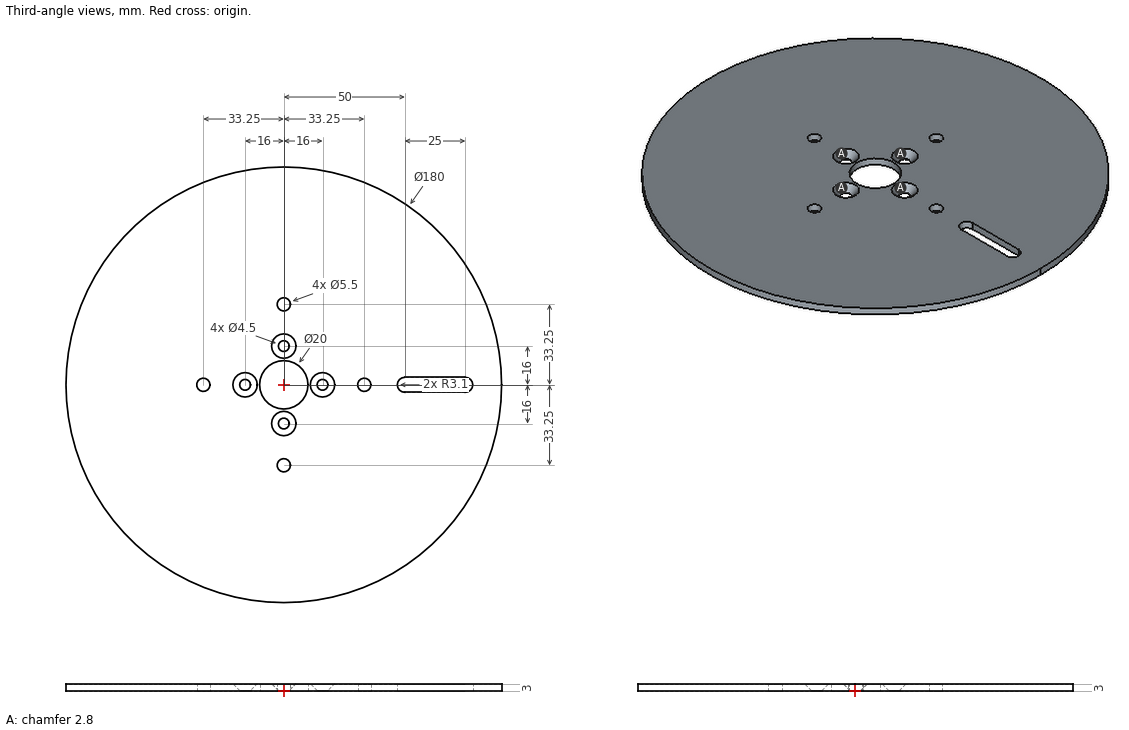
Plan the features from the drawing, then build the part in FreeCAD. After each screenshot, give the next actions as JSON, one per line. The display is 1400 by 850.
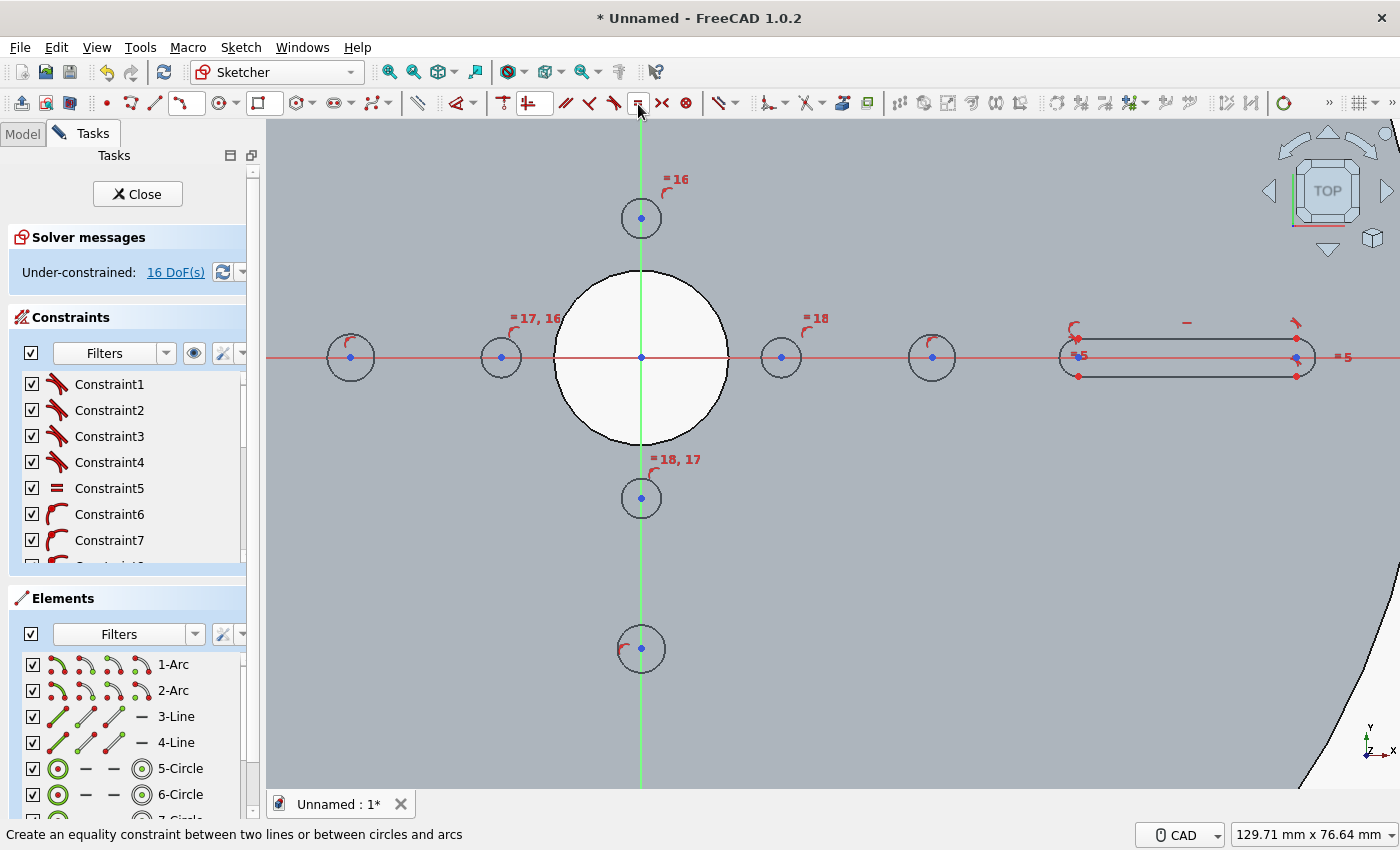
{"action": "scroll", "coordinate": [641, 650], "scroll_direction": "down", "scroll_amount": 2}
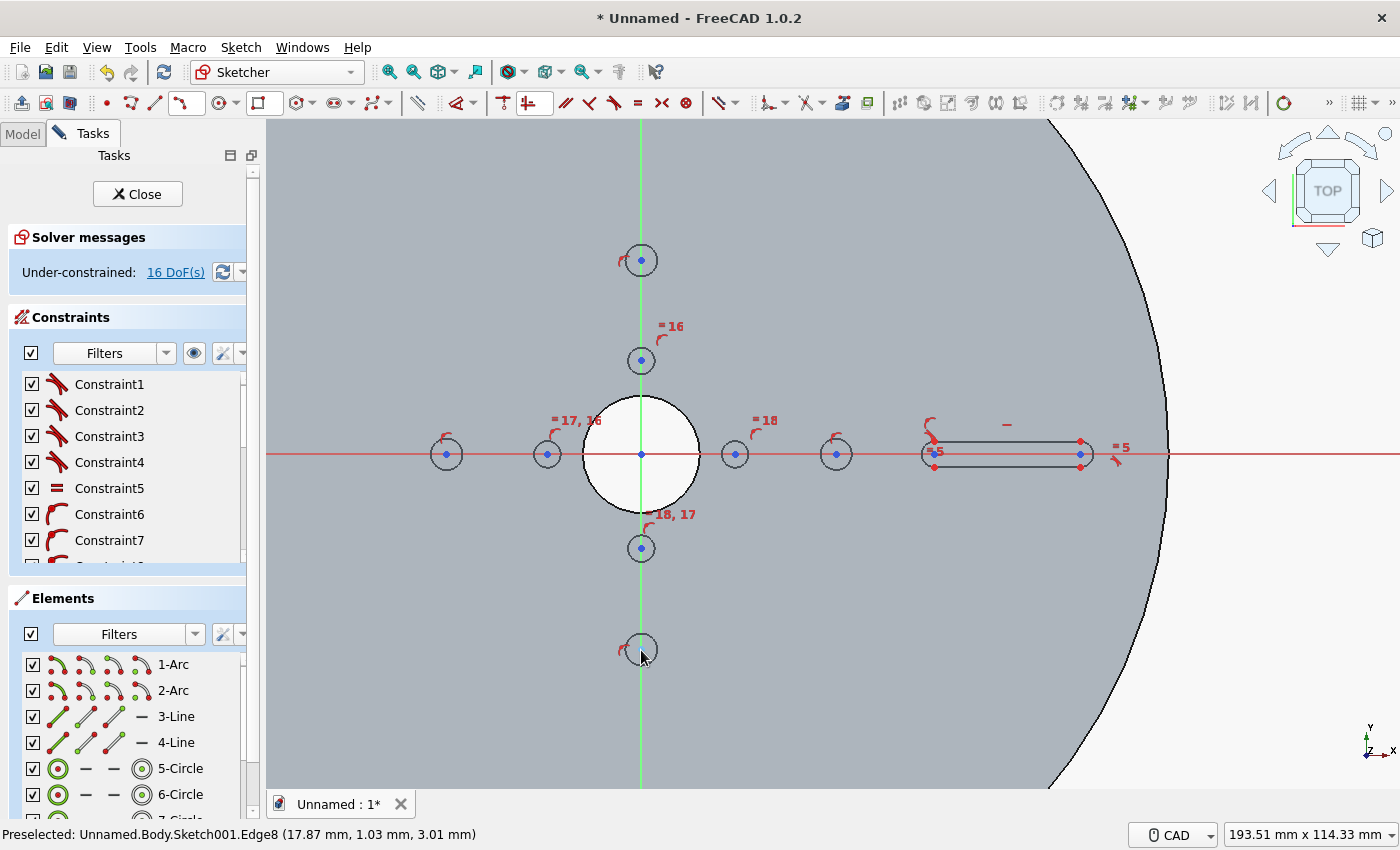
{"action": "scroll", "coordinate": [653, 249], "scroll_direction": "up", "scroll_amount": 2}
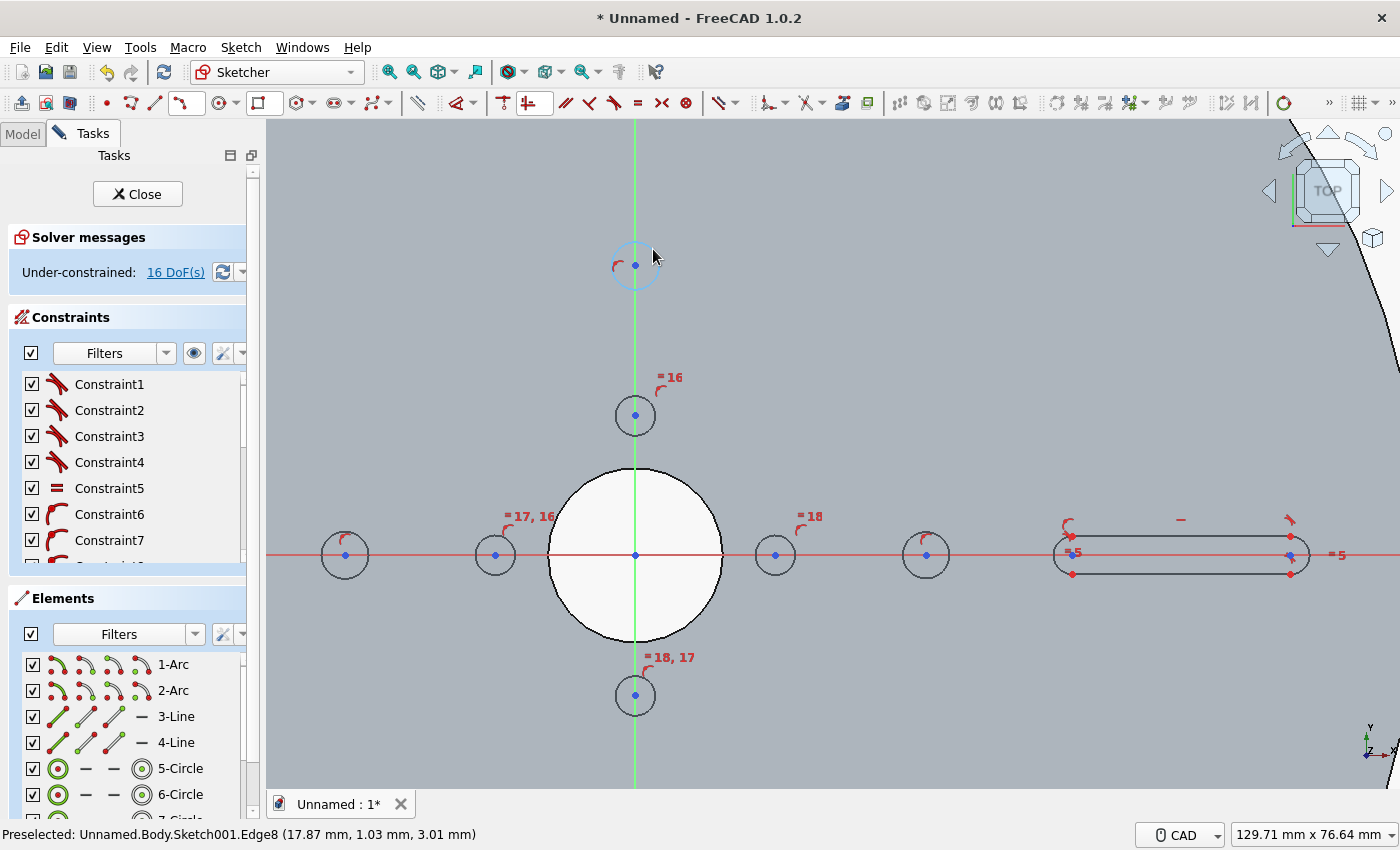
{"action": "left_click", "coordinate": [652, 249]}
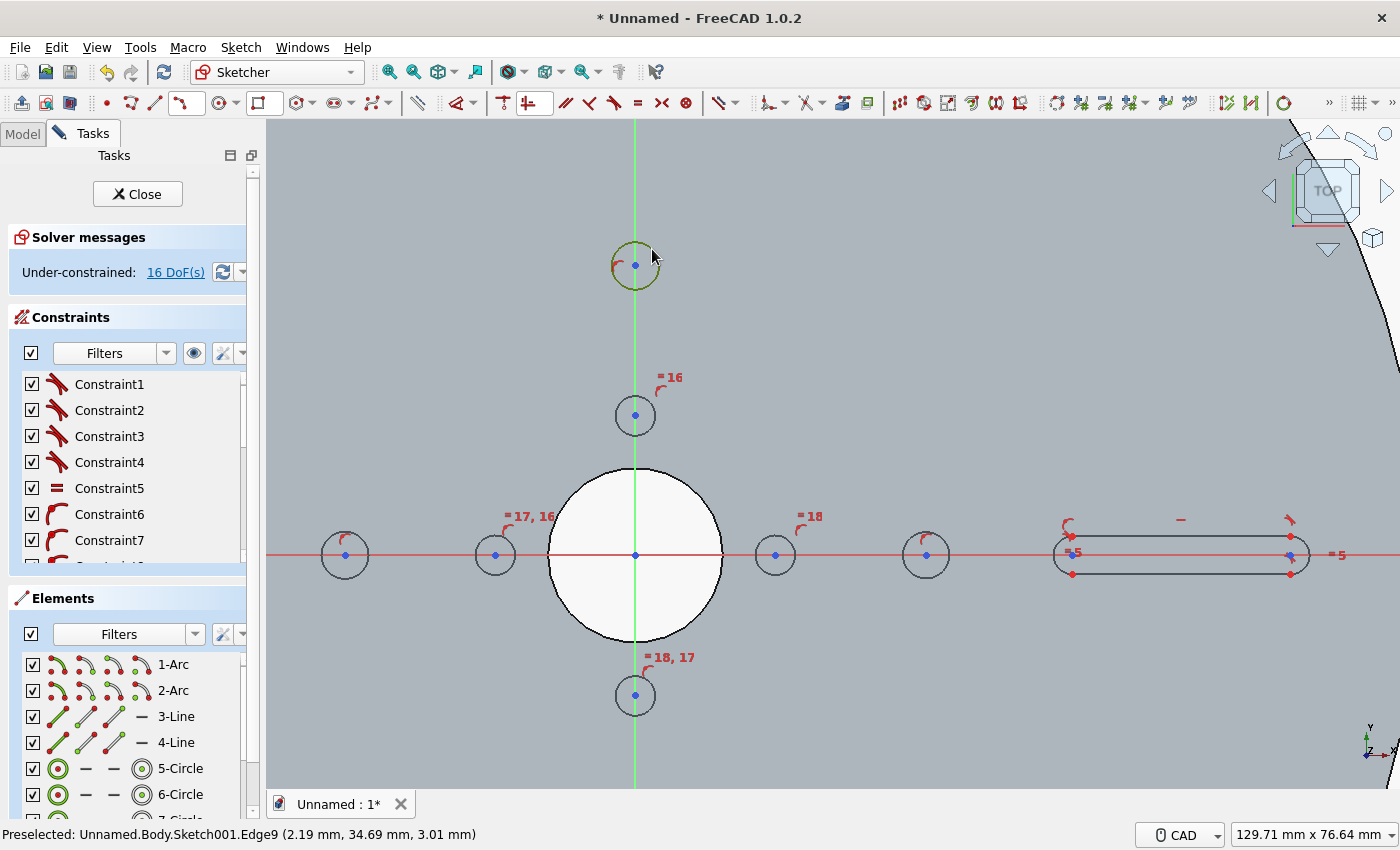
{"action": "left_click", "coordinate": [362, 539]}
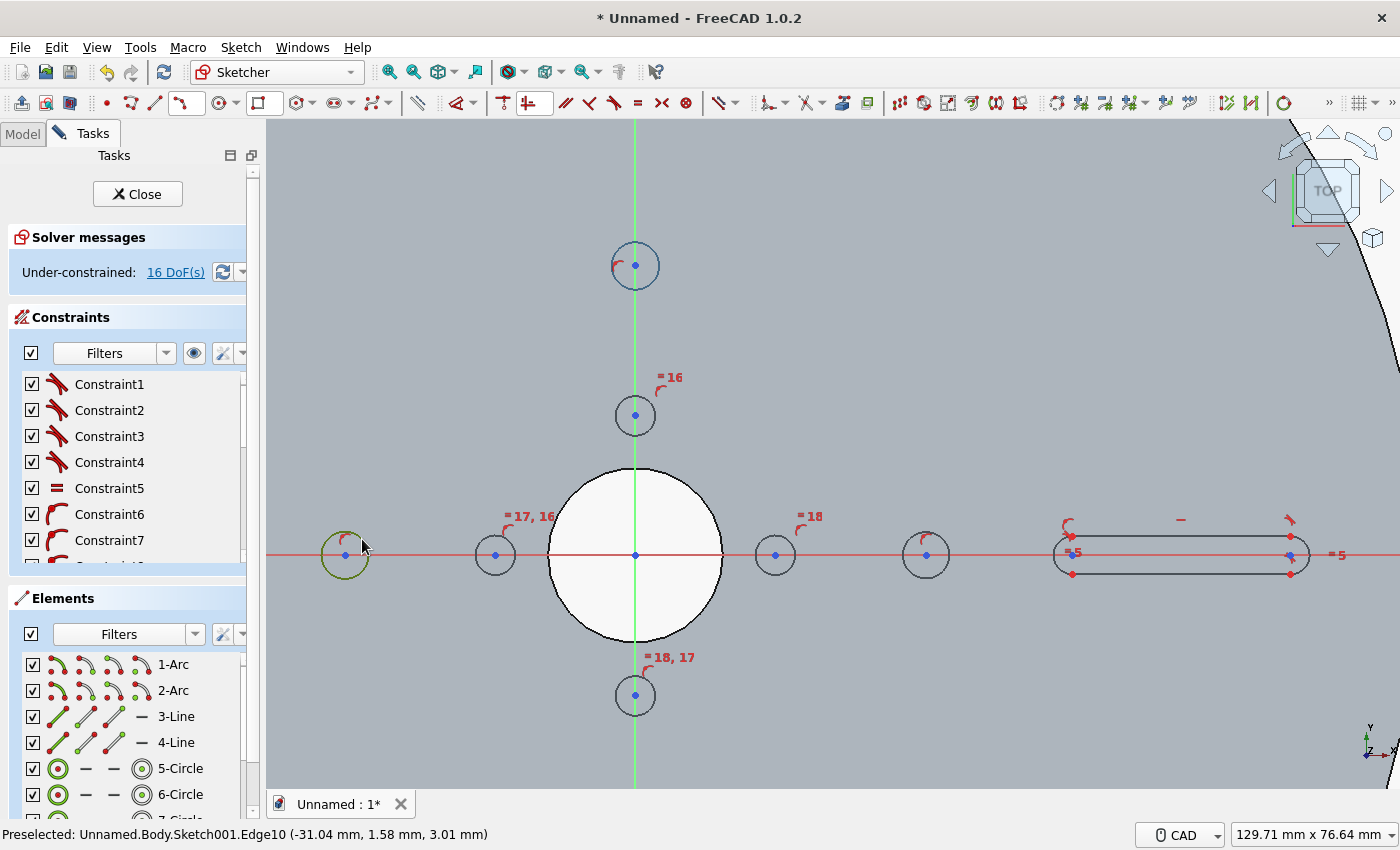
{"action": "scroll", "coordinate": [653, 248], "scroll_direction": "down", "scroll_amount": 2}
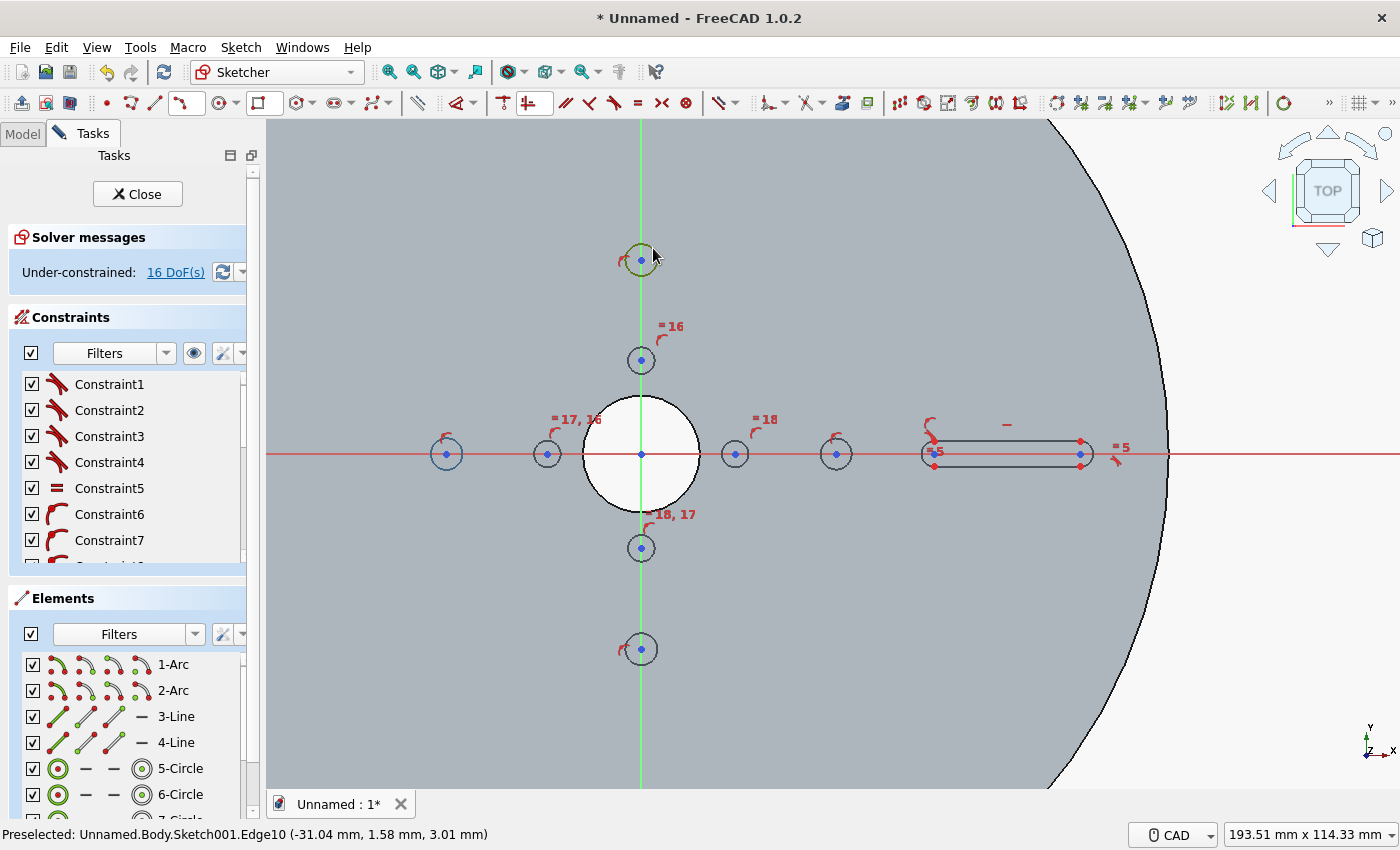
{"action": "scroll", "coordinate": [653, 638], "scroll_direction": "up", "scroll_amount": 2}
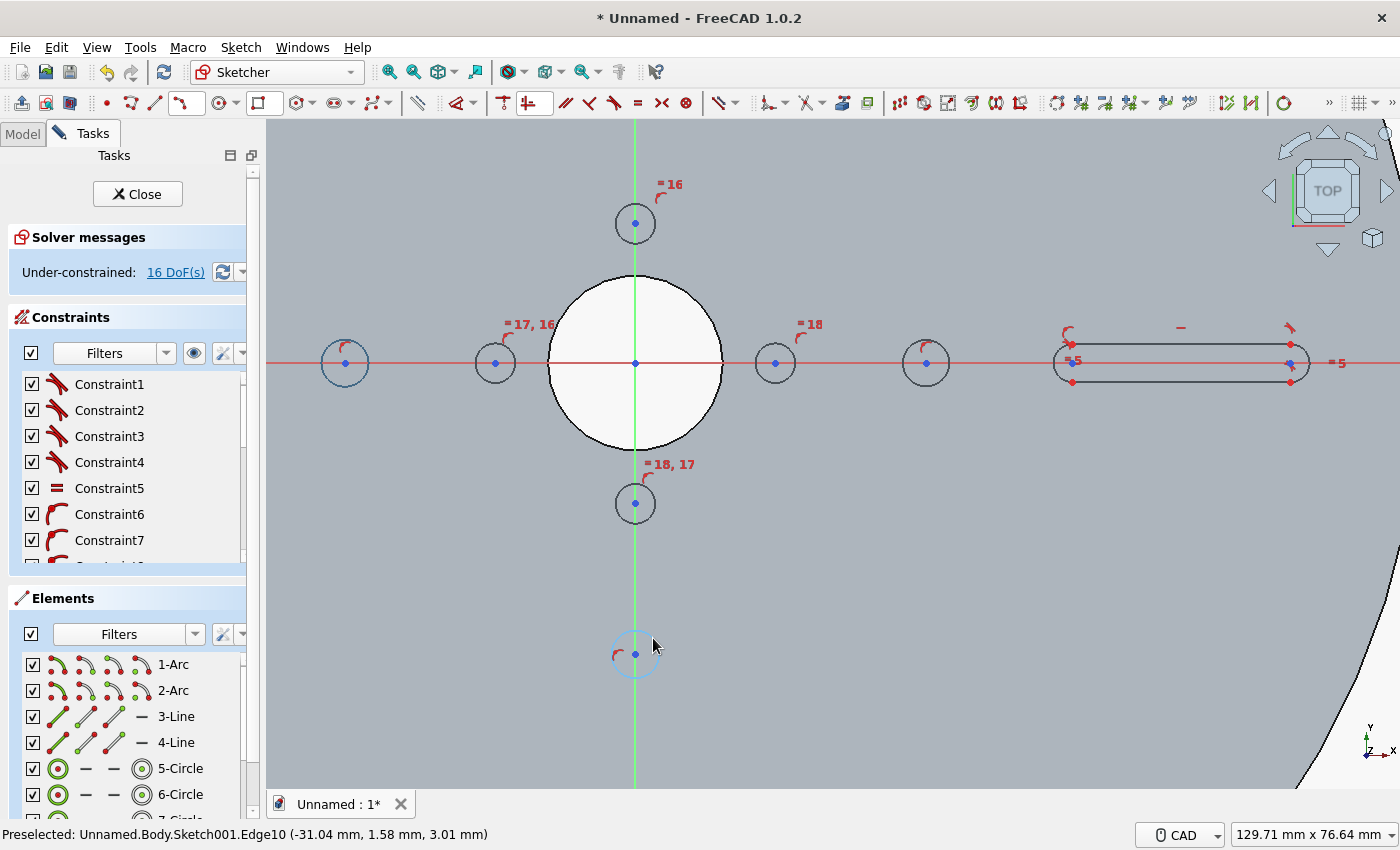
{"action": "left_click", "coordinate": [652, 638]}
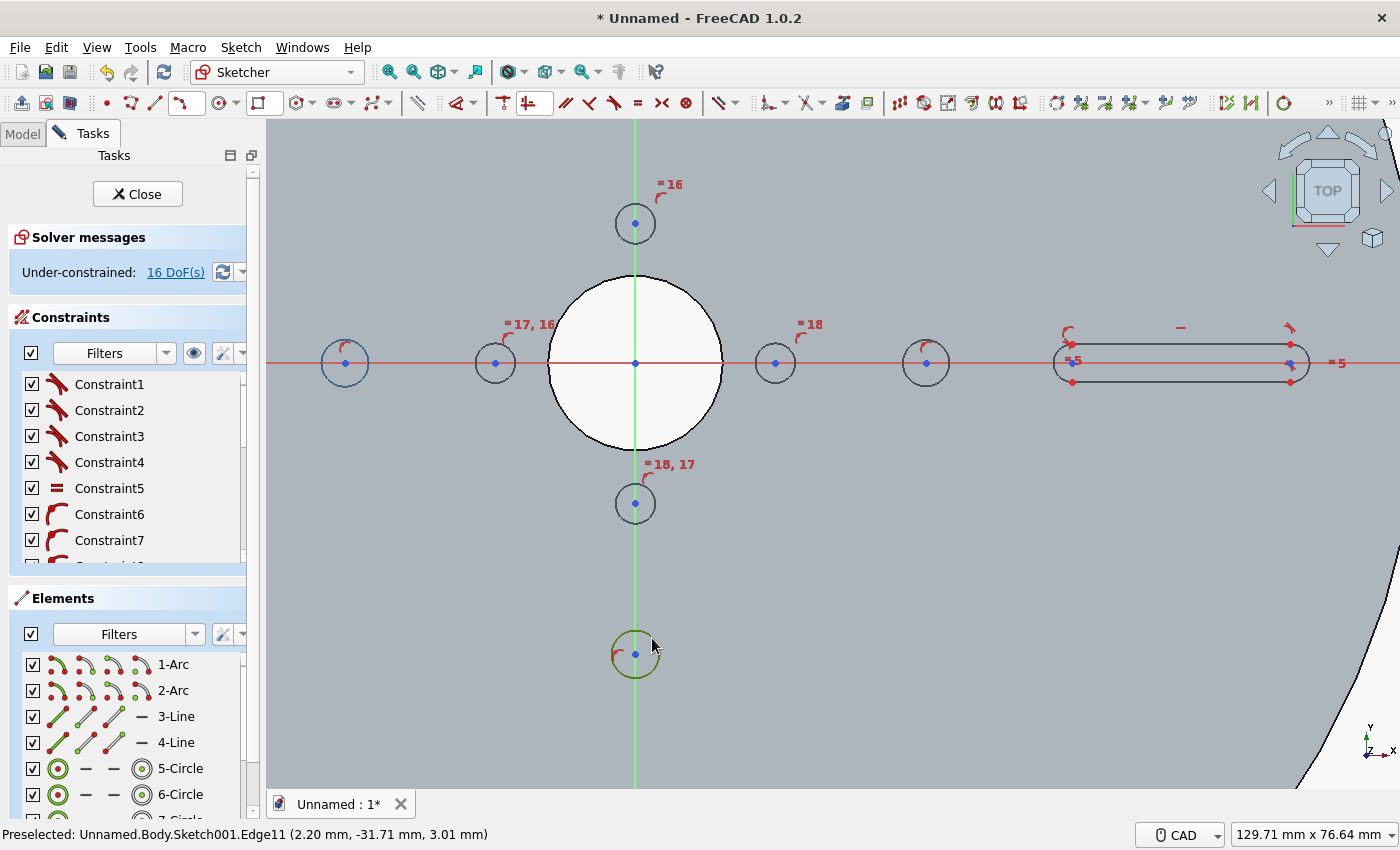
{"action": "left_click", "coordinate": [942, 347]}